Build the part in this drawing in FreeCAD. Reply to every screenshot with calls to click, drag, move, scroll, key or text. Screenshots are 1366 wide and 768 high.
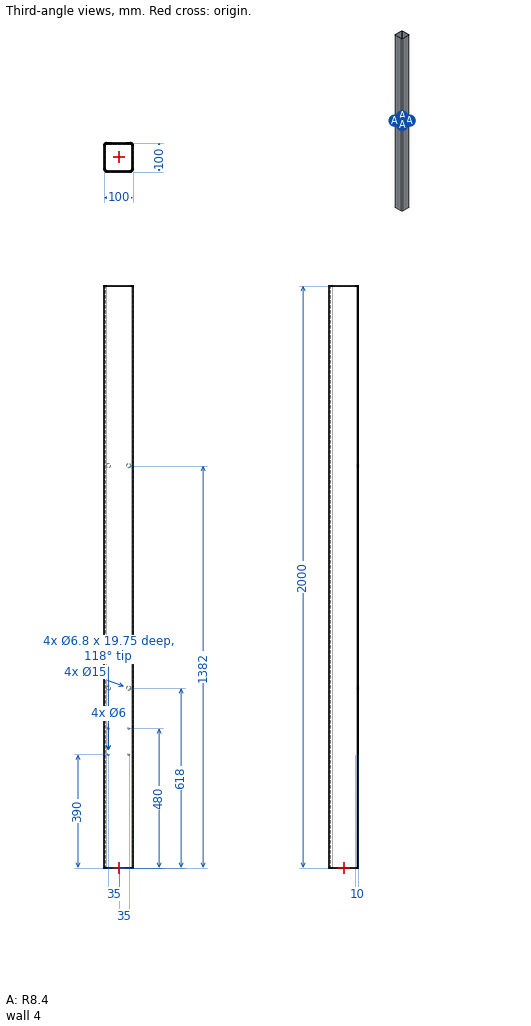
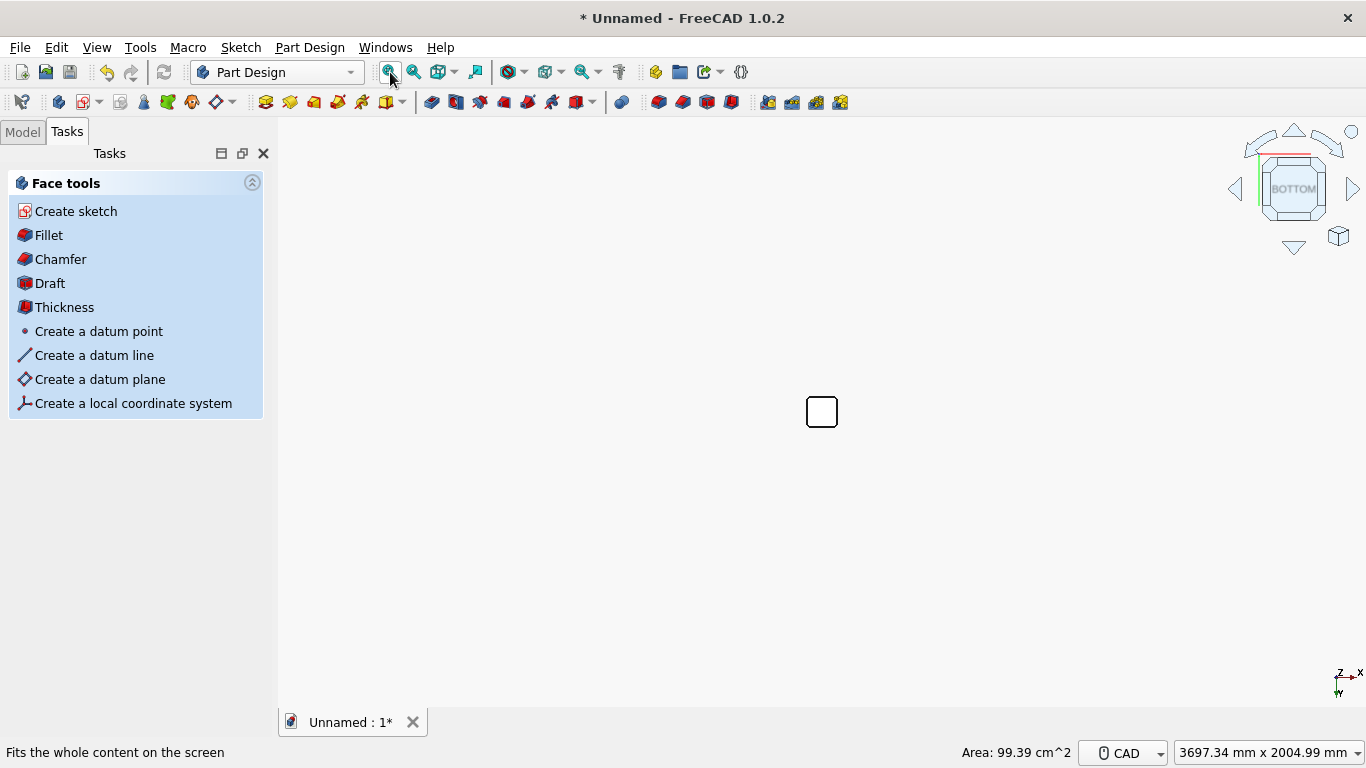
click(390, 72)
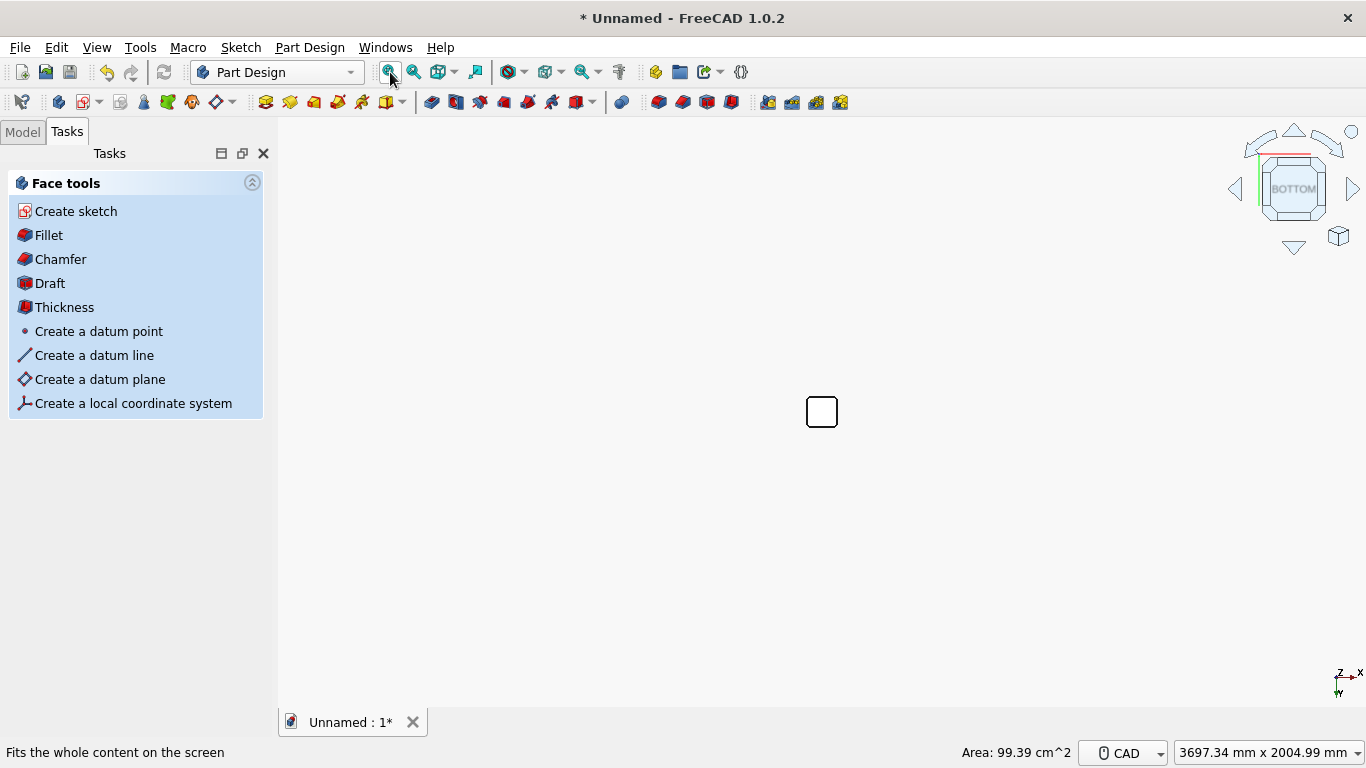
click(822, 411, ctrl)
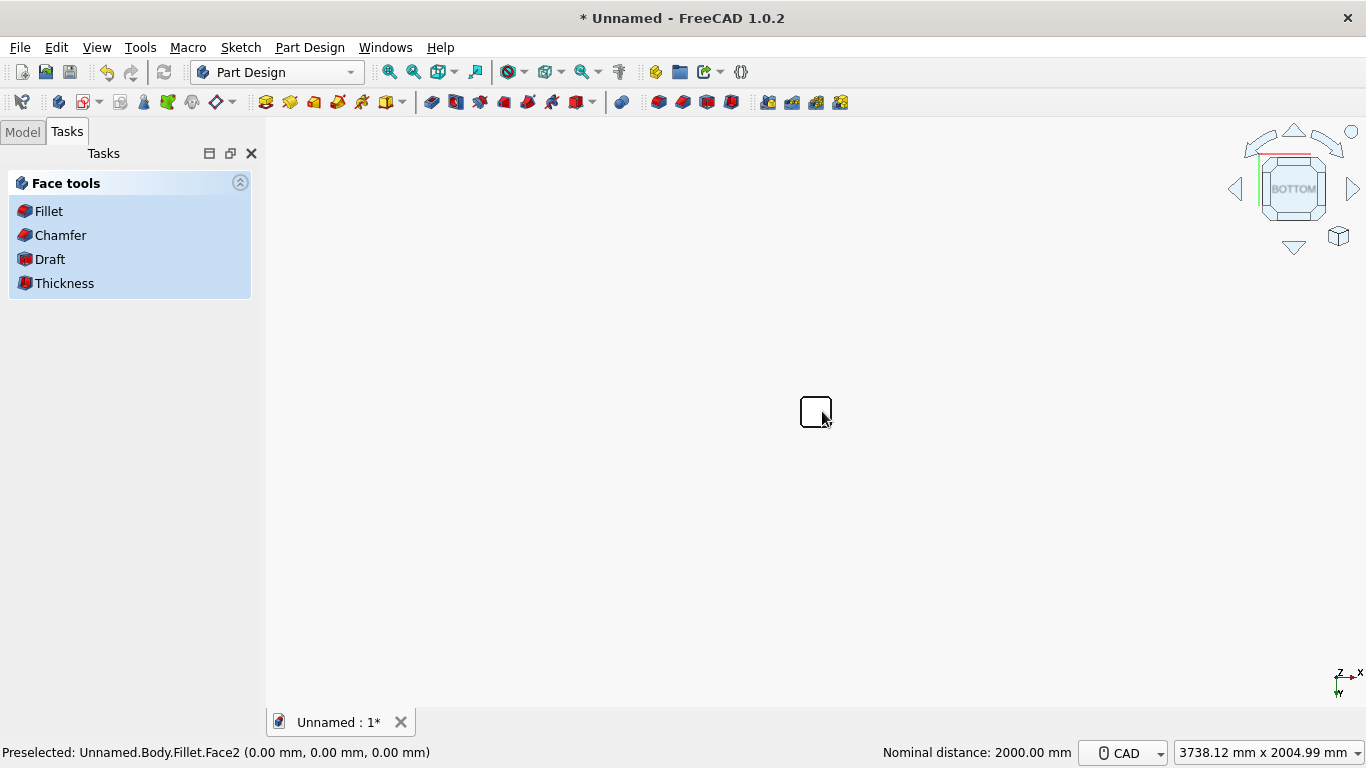
click(732, 102)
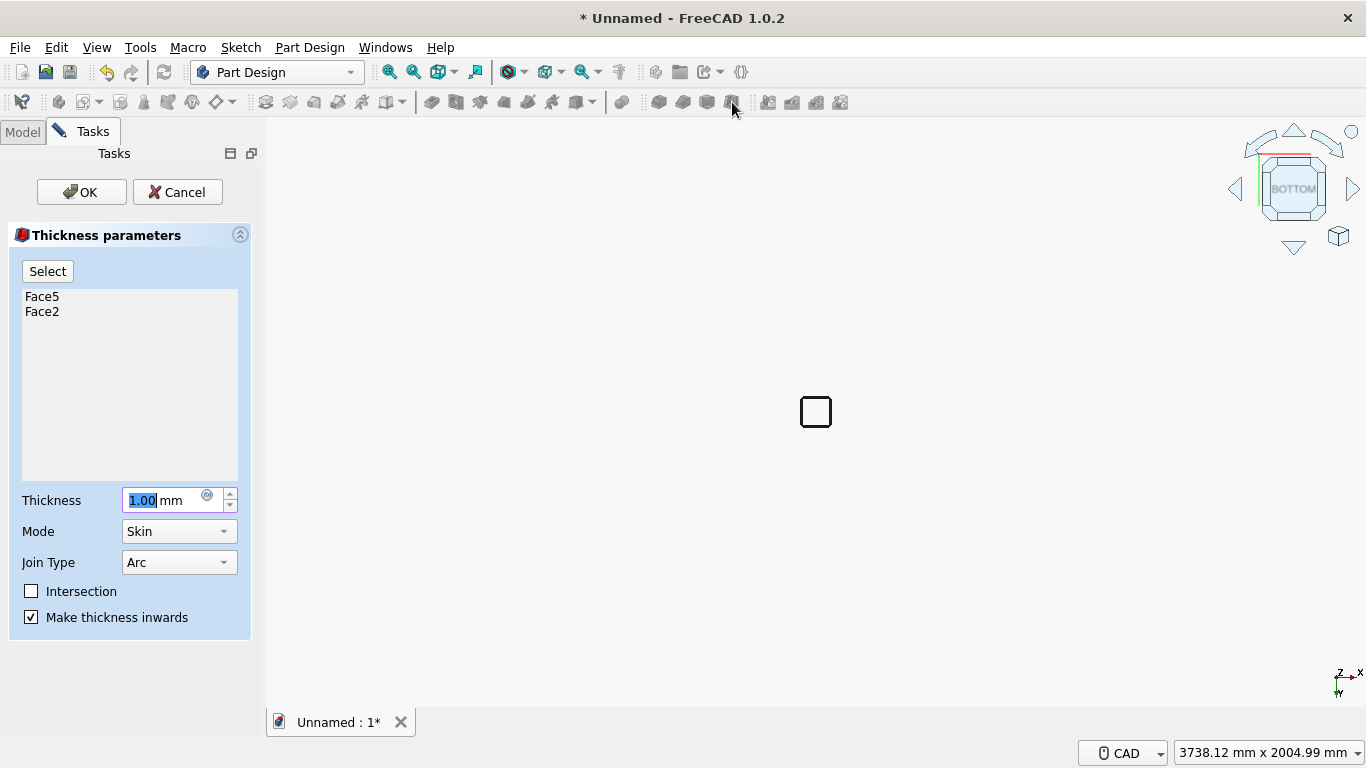
text(4)
key(Tab)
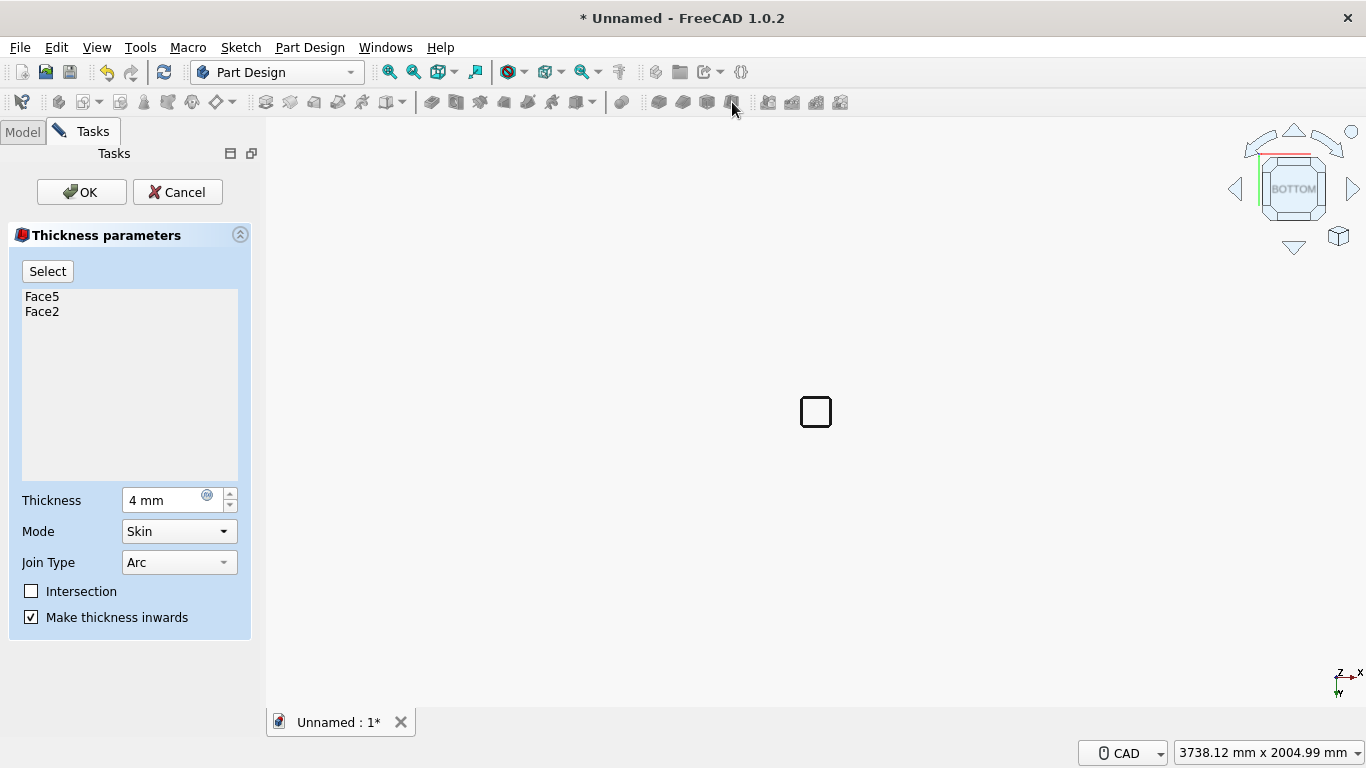
click(180, 562)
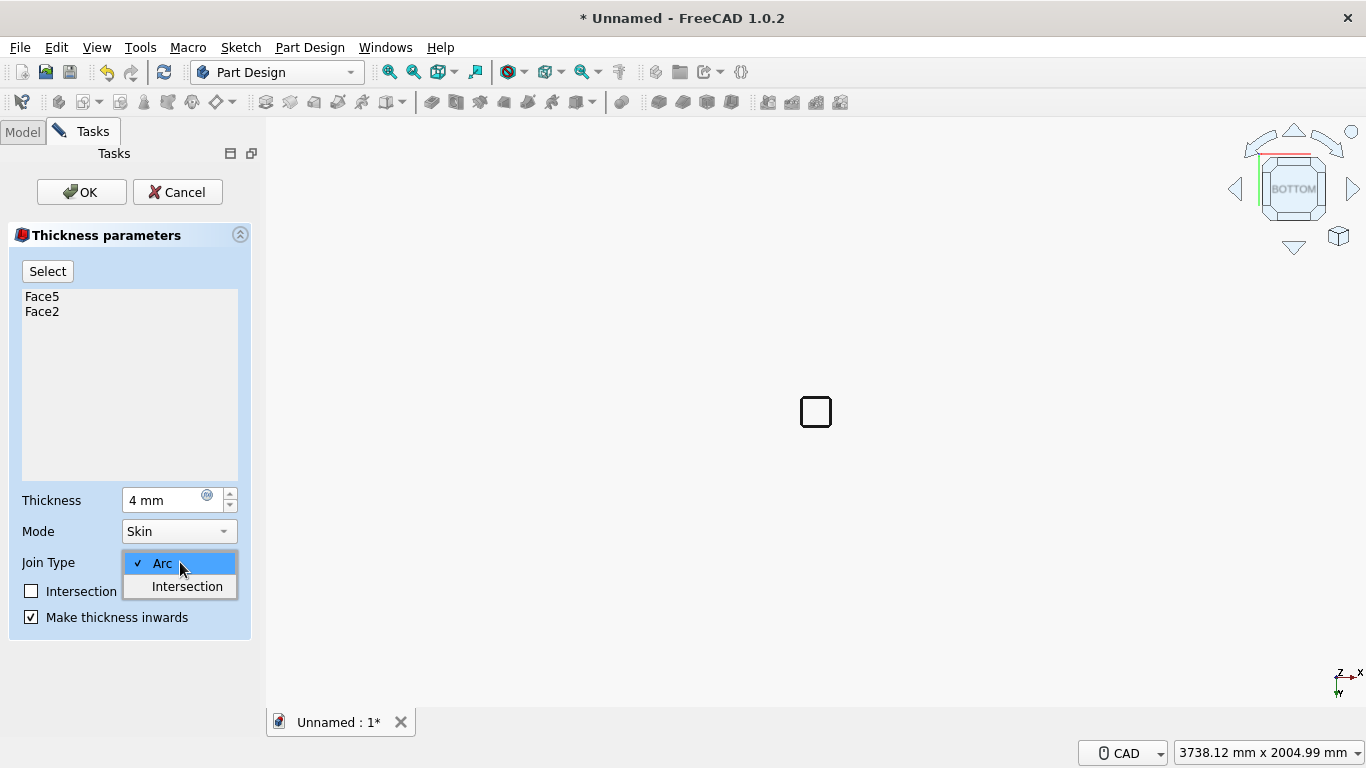
click(179, 586)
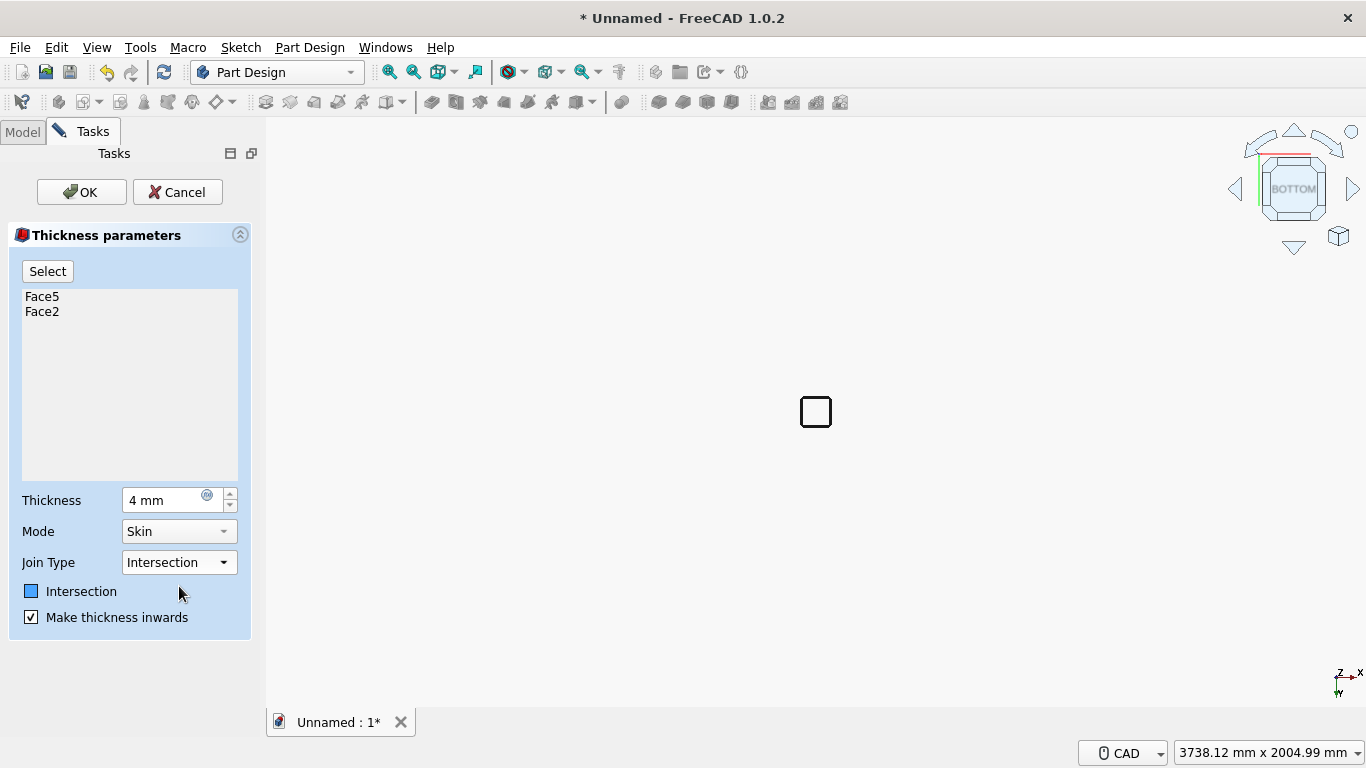
click(82, 192)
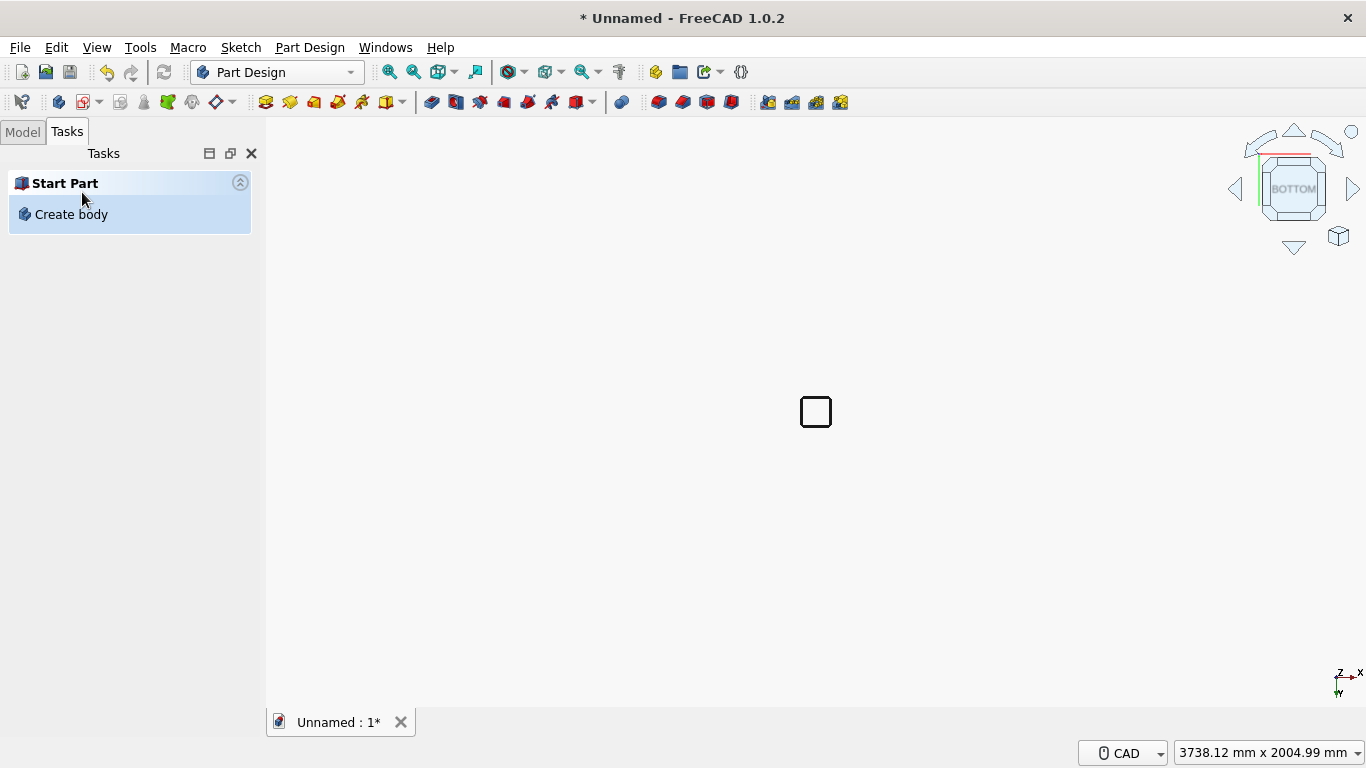
click(390, 72)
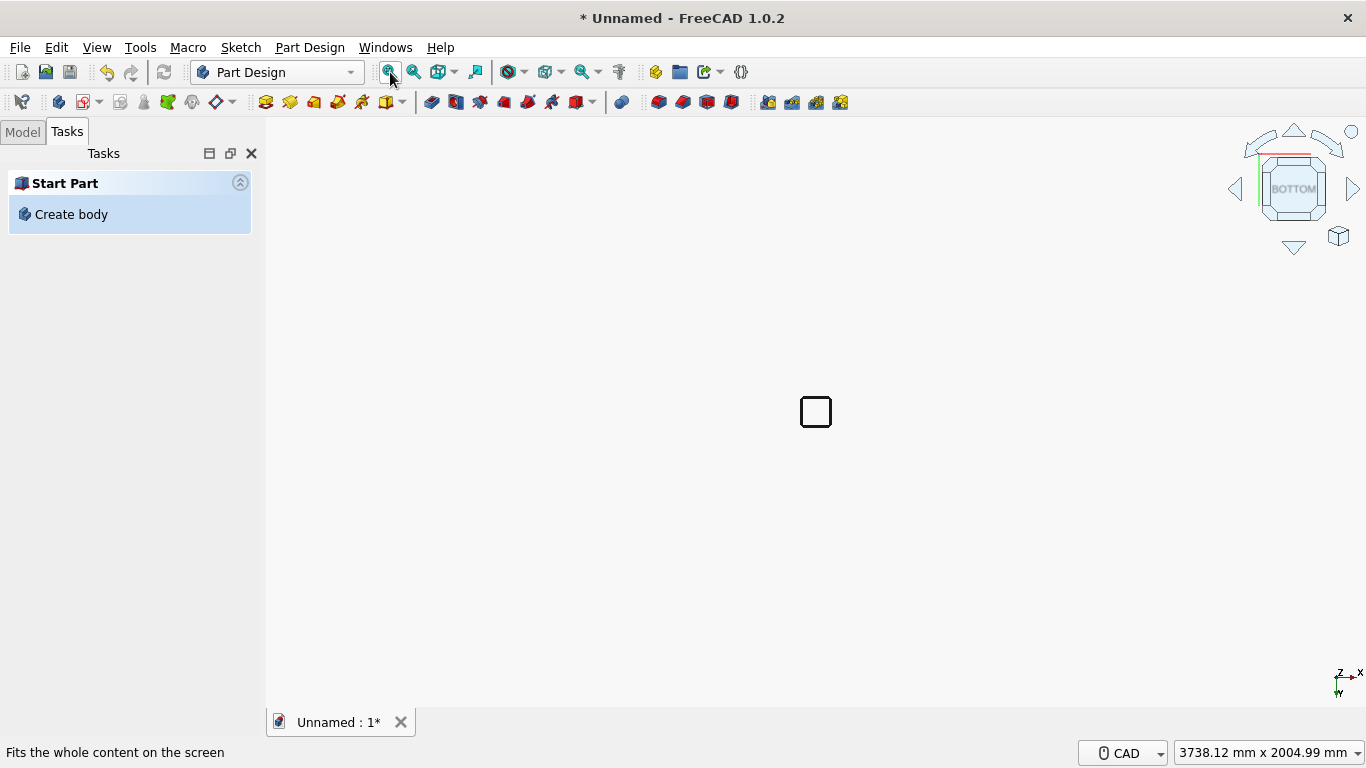
key(4)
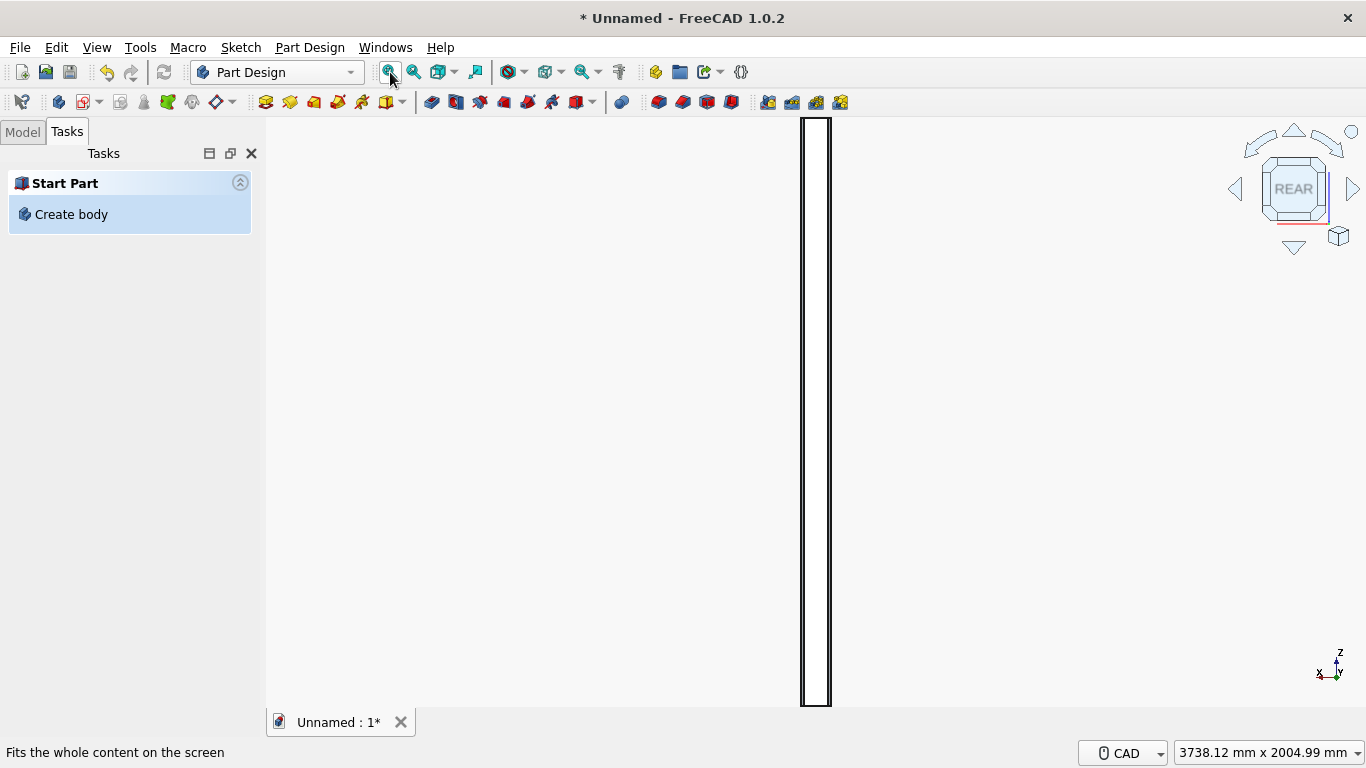
click(816, 159)